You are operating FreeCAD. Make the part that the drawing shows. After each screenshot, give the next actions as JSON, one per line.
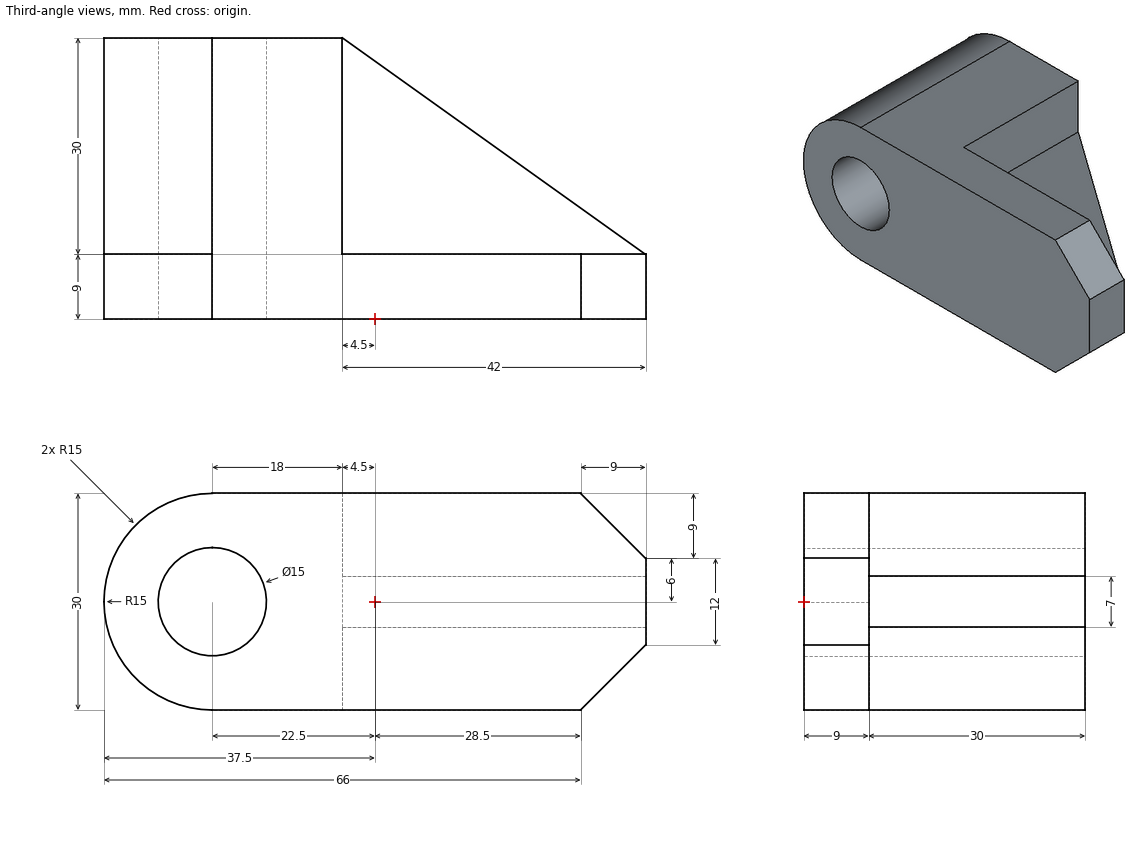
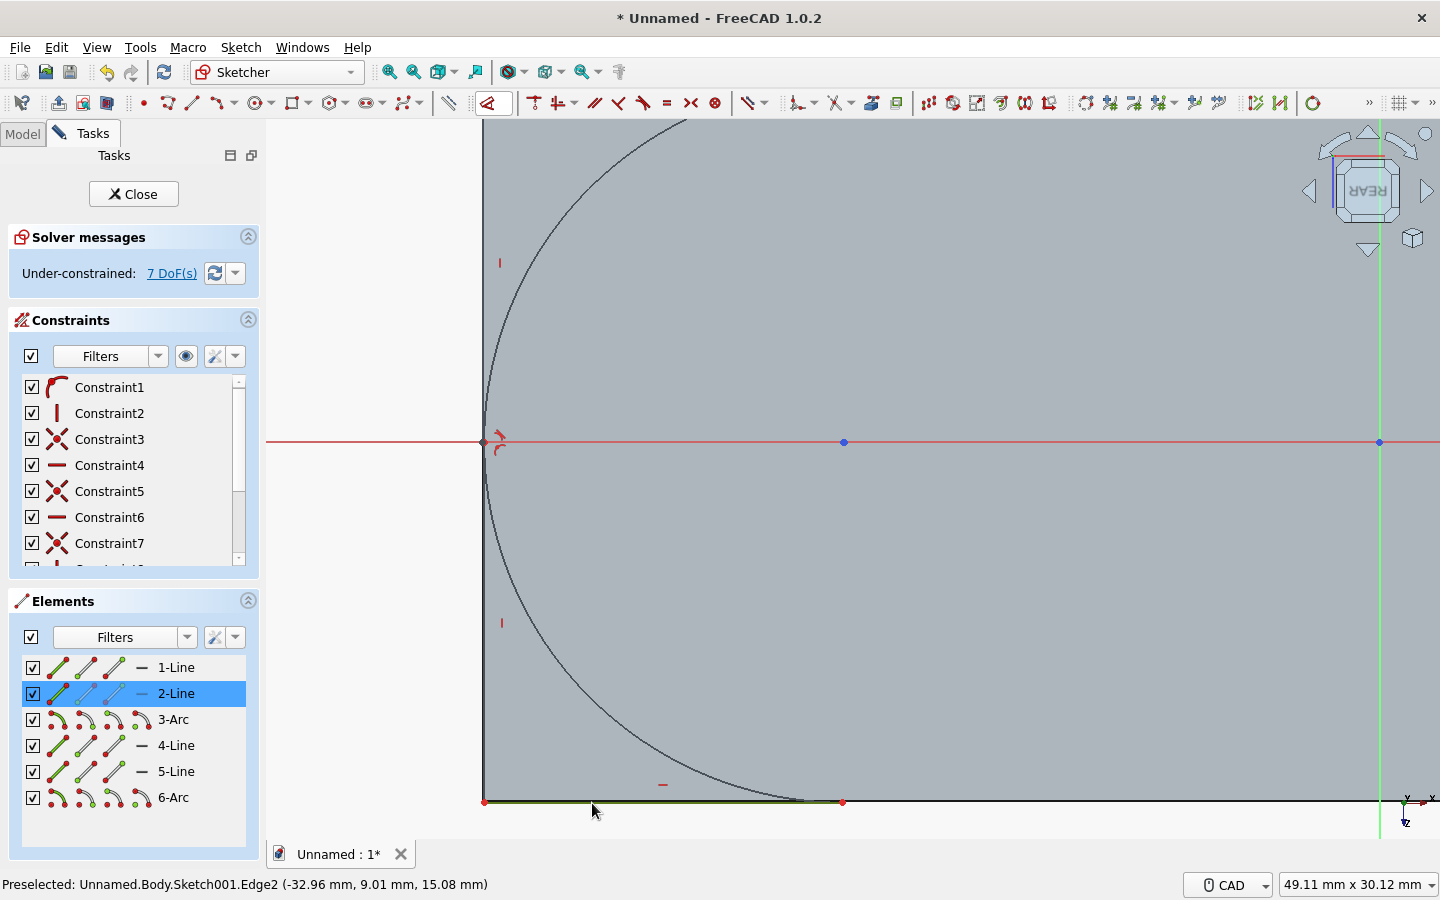
{"action": "left_click", "coordinate": [523, 605]}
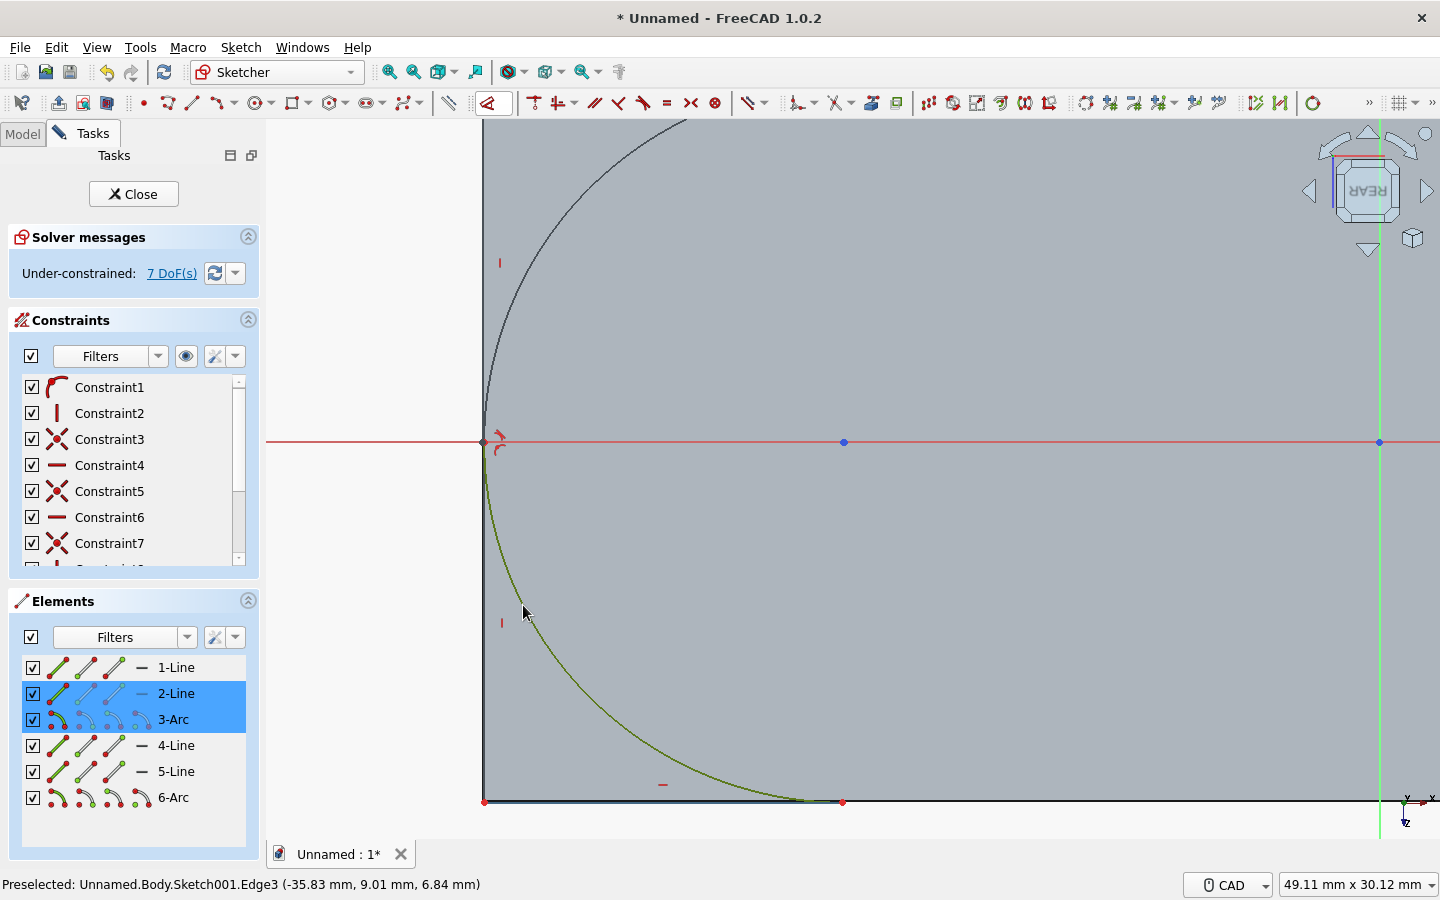
{"action": "key", "text": "t"}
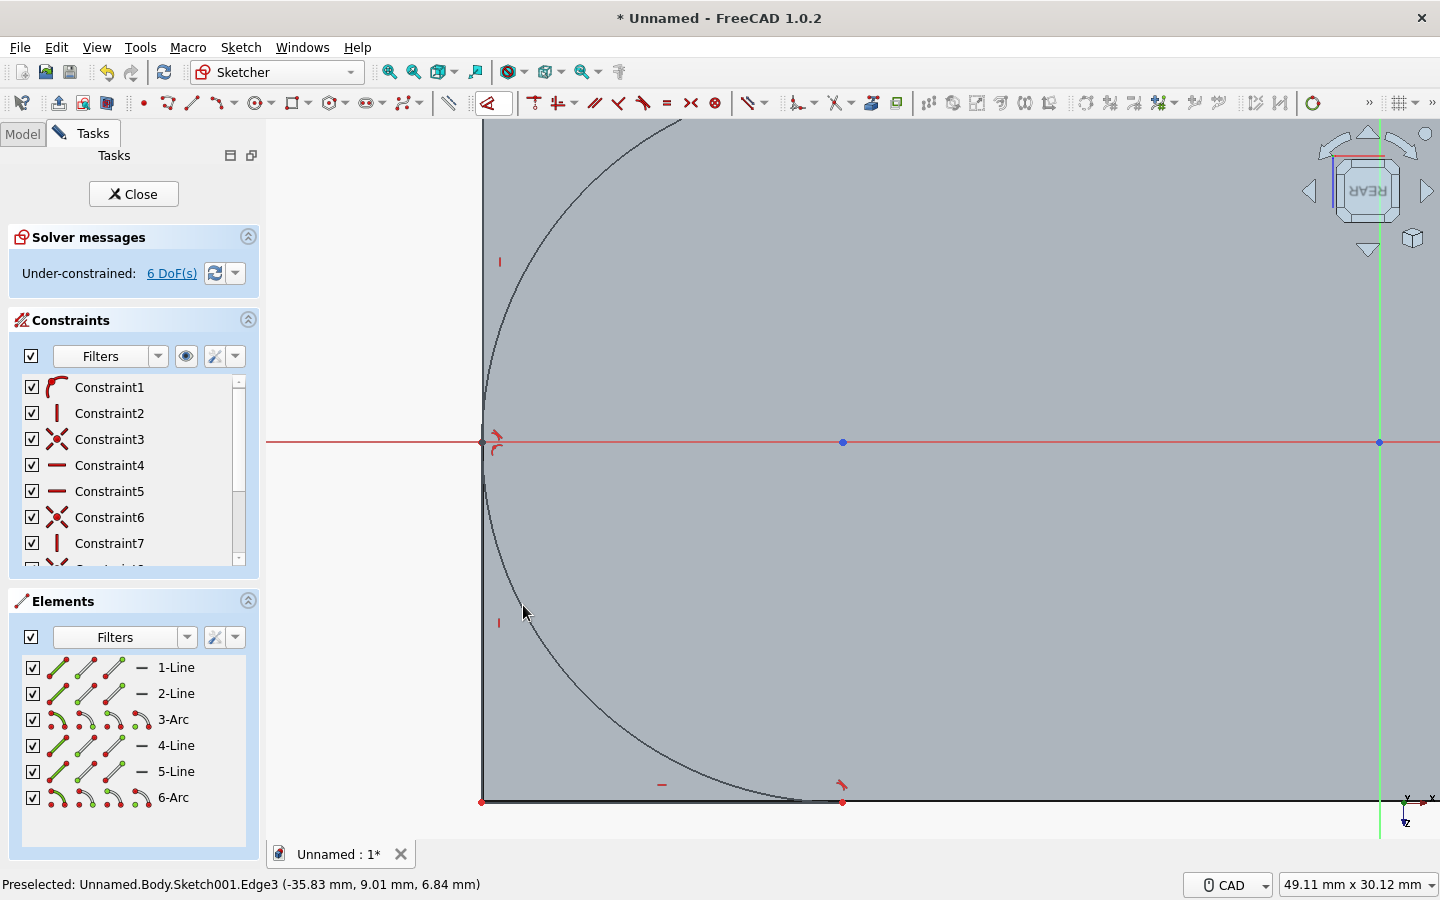
{"action": "left_click", "coordinate": [521, 606]}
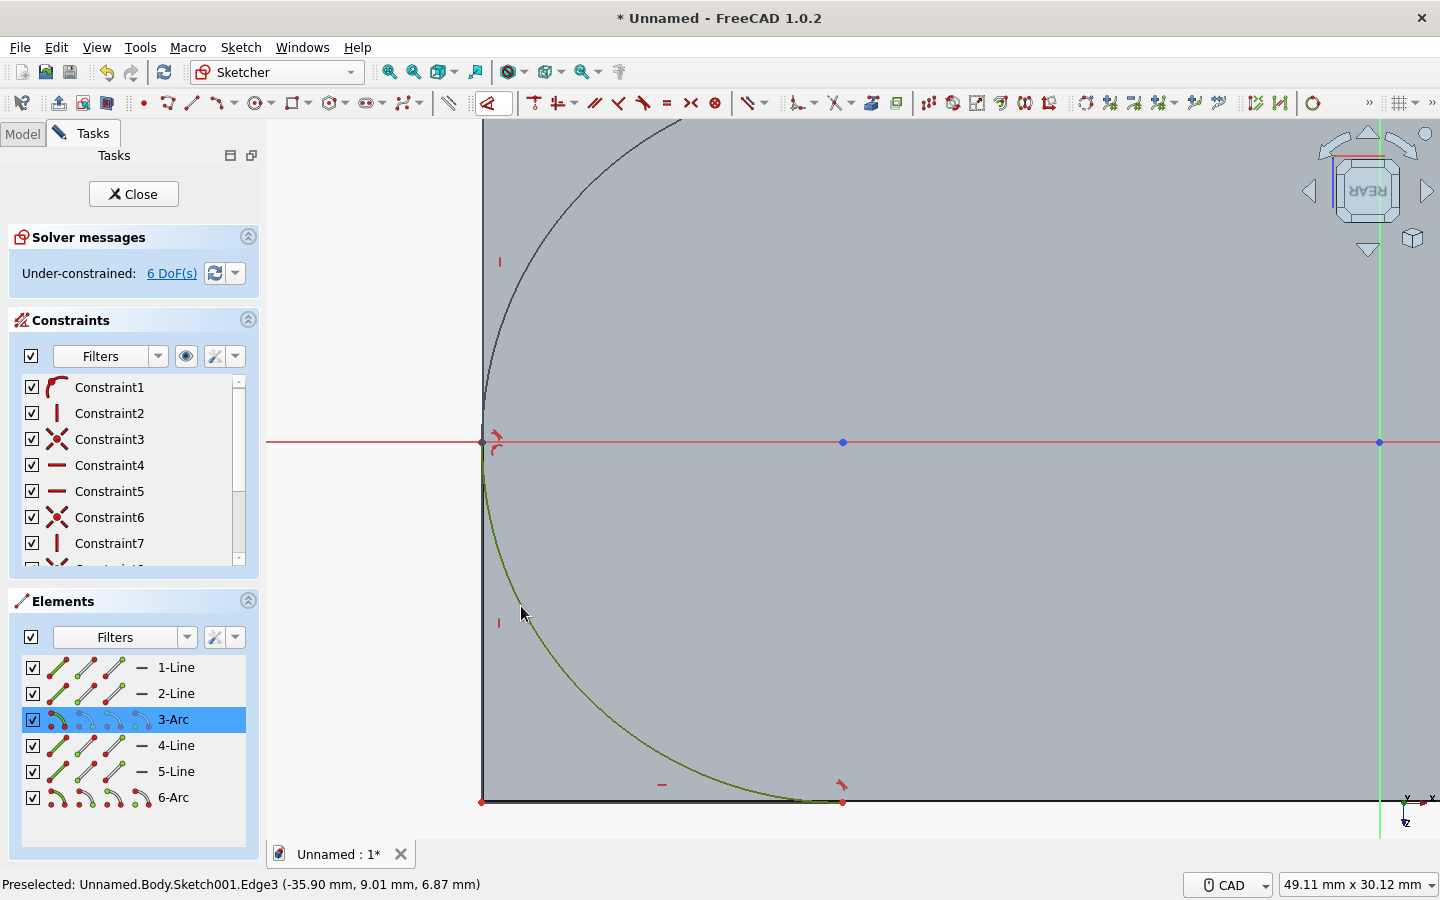
{"action": "left_click", "coordinate": [483, 190]}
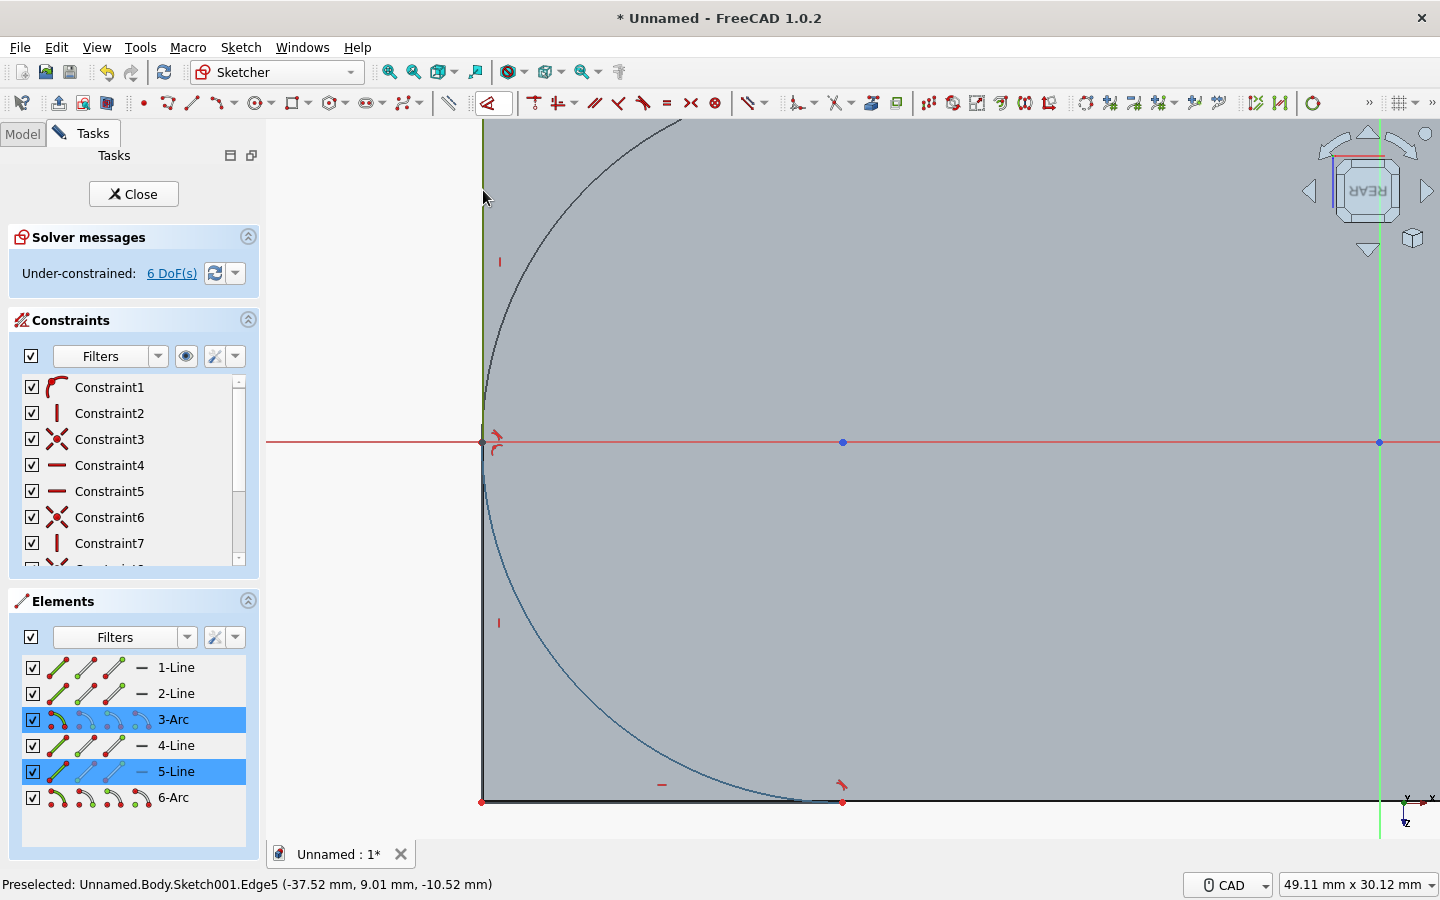
{"action": "left_click", "coordinate": [644, 104]}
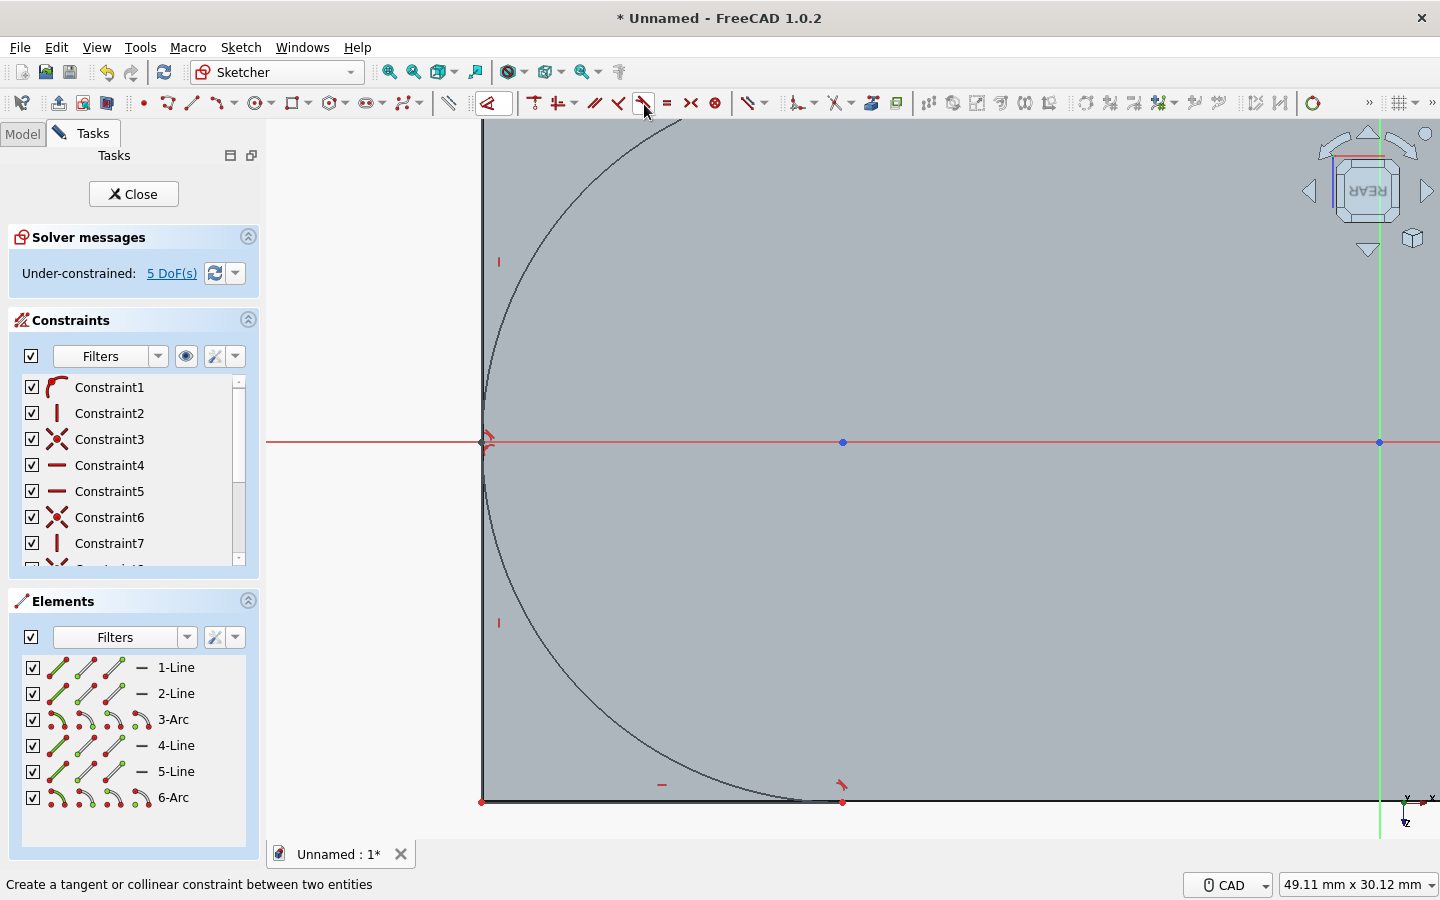
{"action": "scroll", "coordinate": [485, 553], "scroll_direction": "down", "scroll_amount": 2}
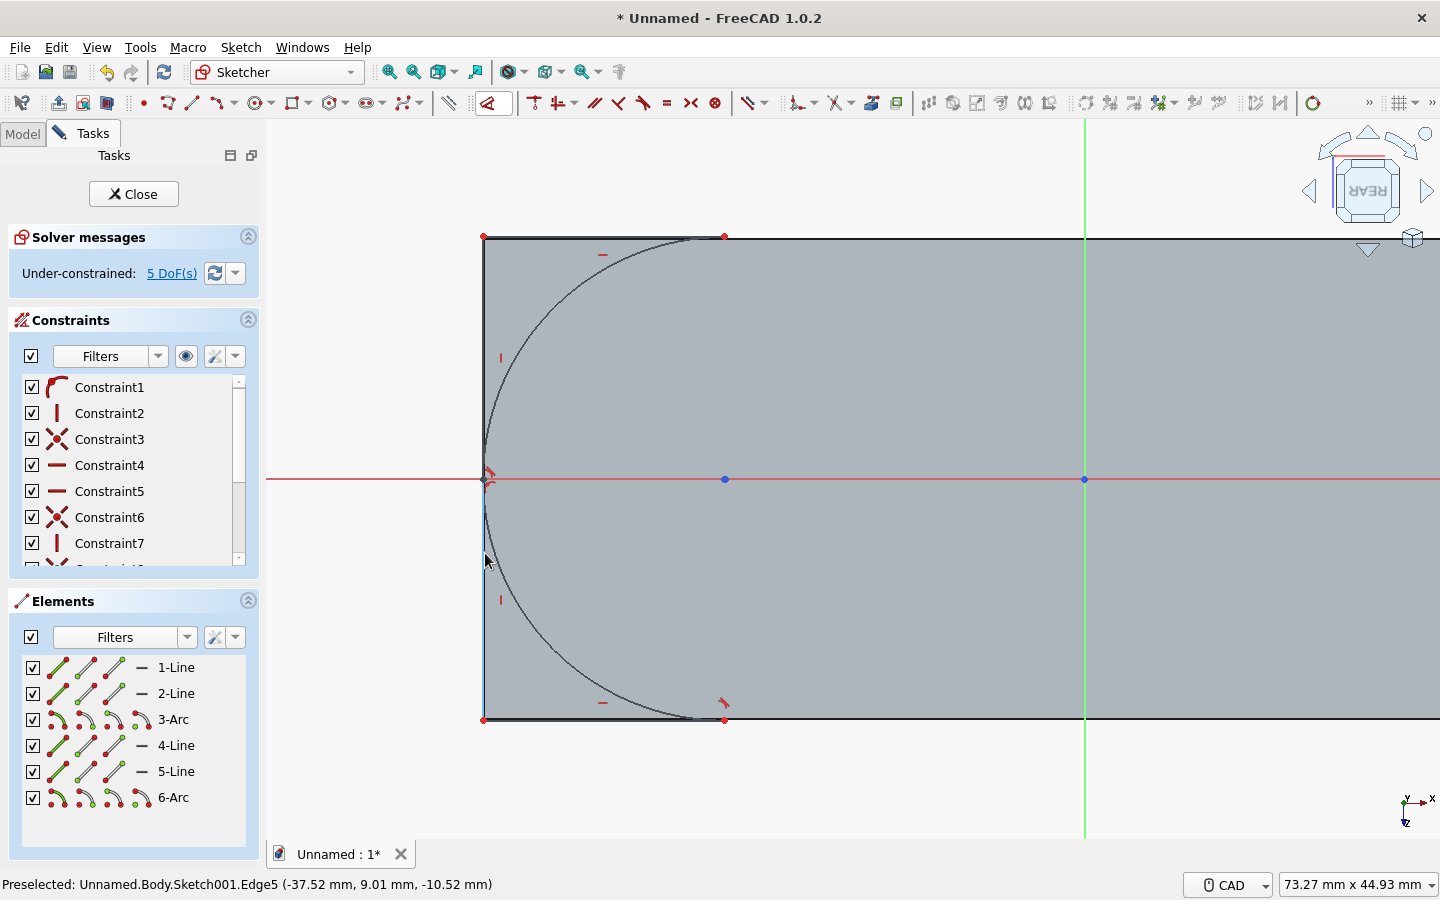
{"action": "scroll", "coordinate": [652, 237], "scroll_direction": "up", "scroll_amount": 2}